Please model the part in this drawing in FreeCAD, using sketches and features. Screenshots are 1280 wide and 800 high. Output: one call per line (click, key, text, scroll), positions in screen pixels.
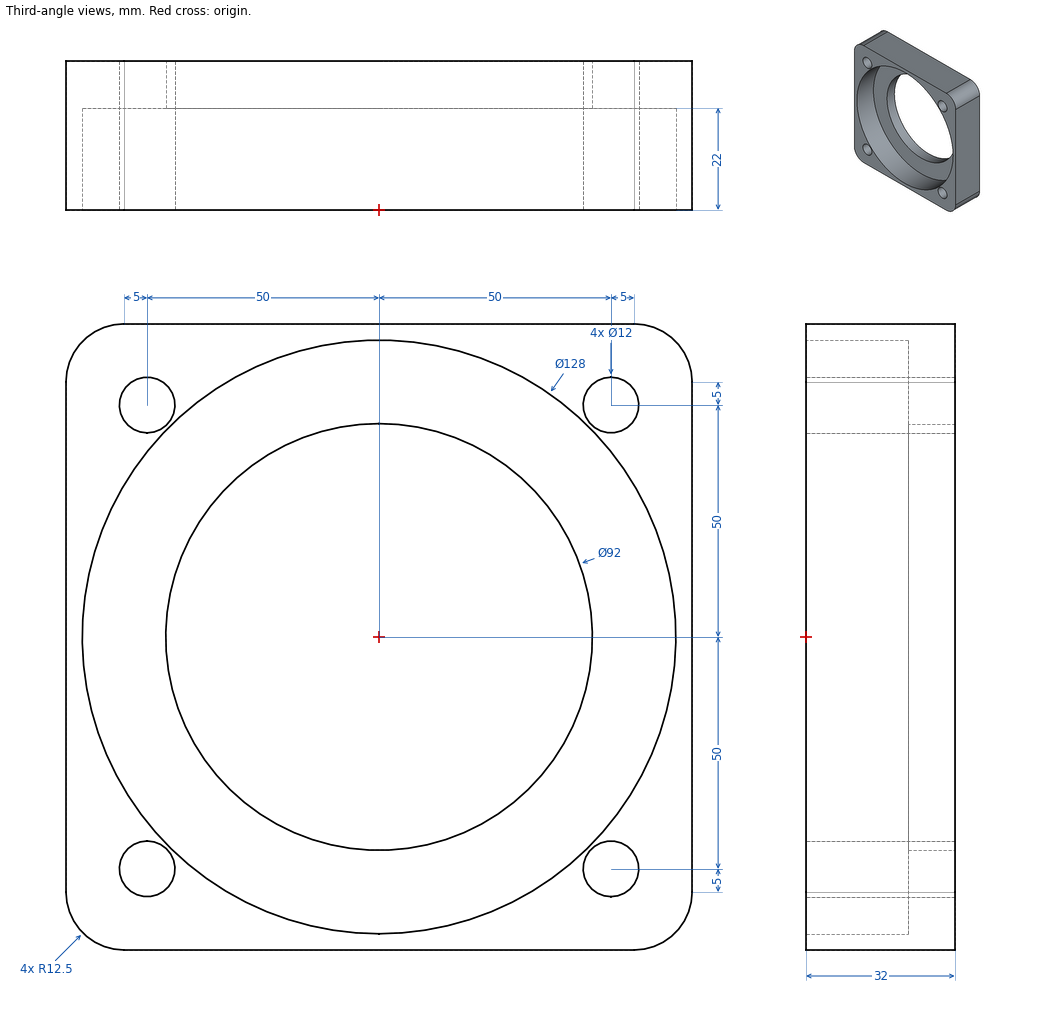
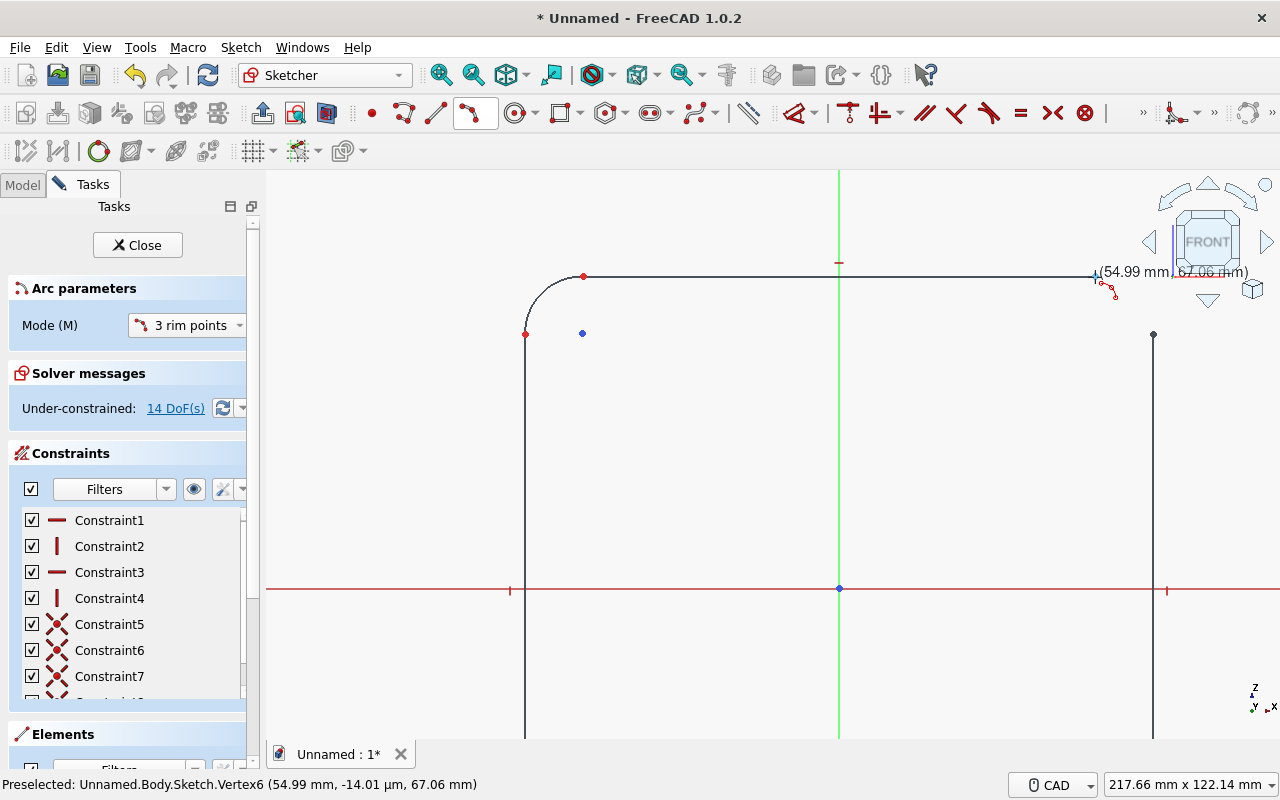
scroll(541, 291, down, 3)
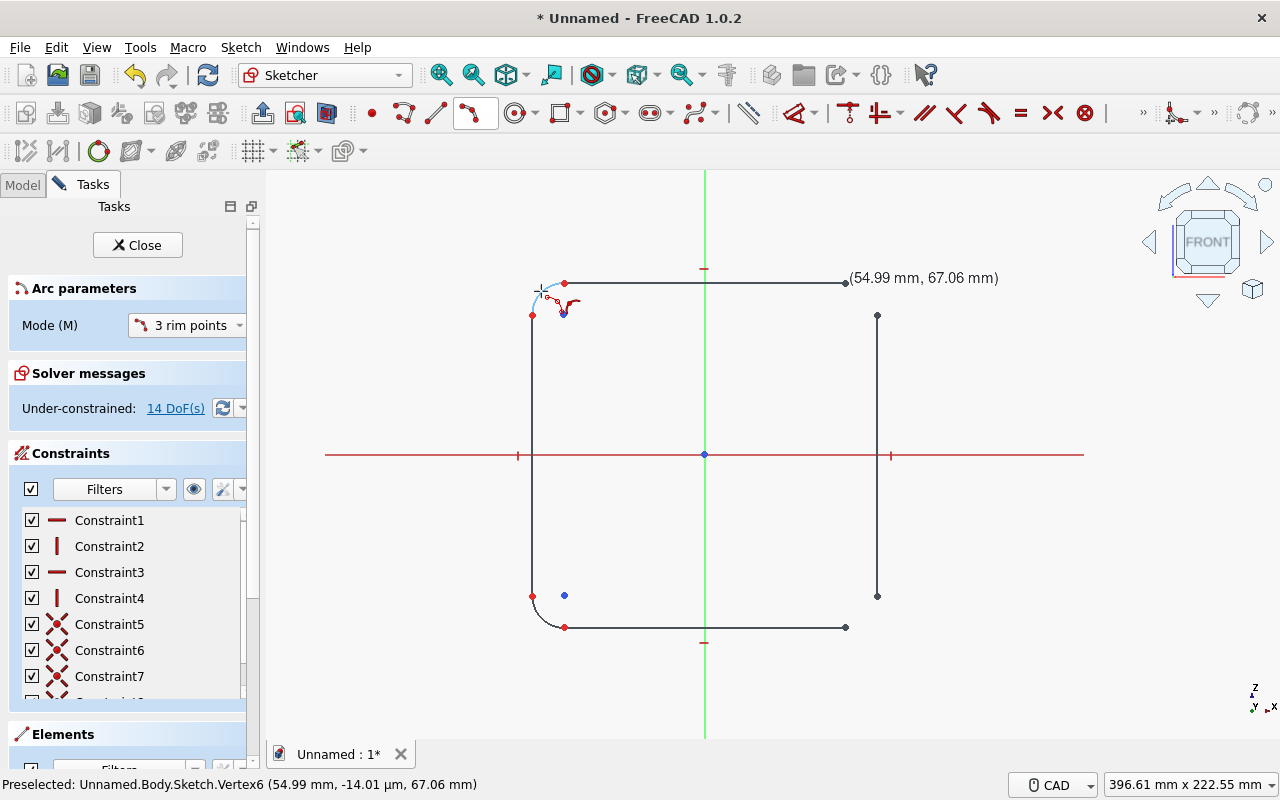
click(877, 315)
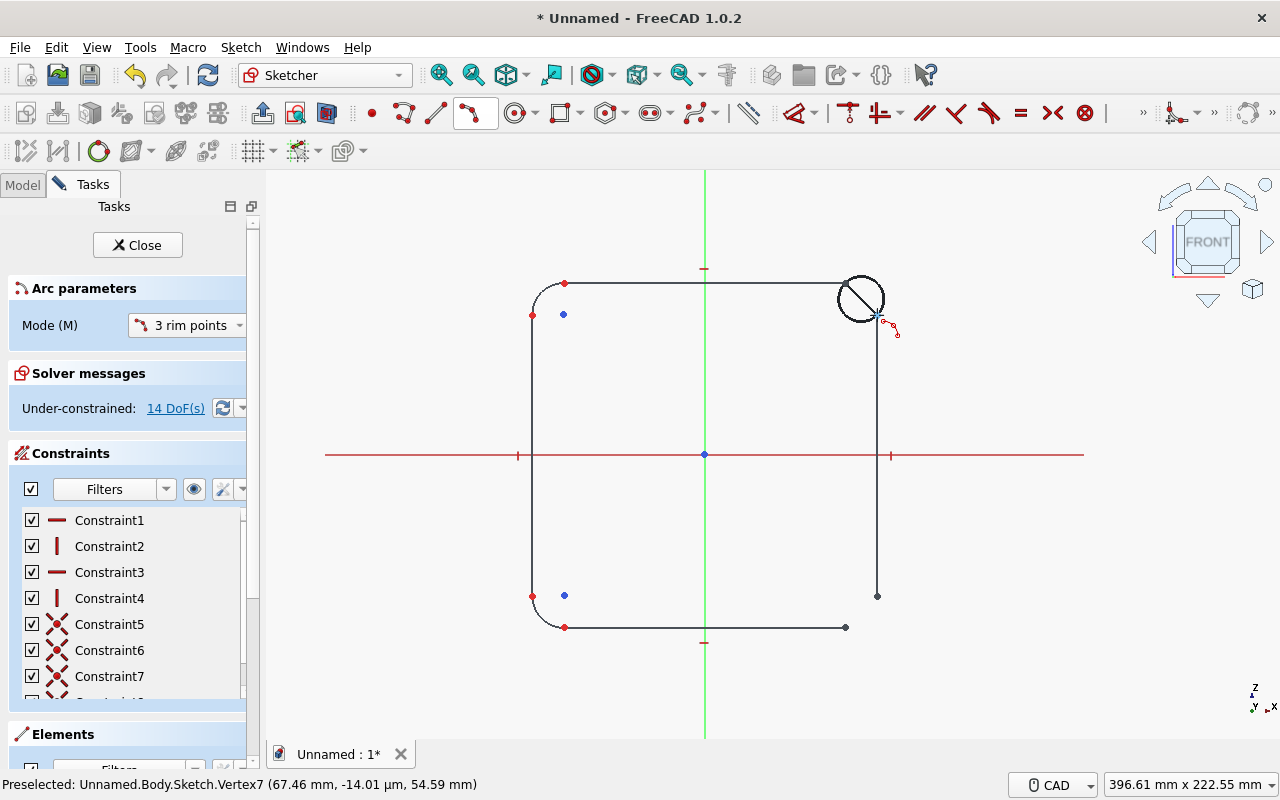
scroll(868, 291, up, 3)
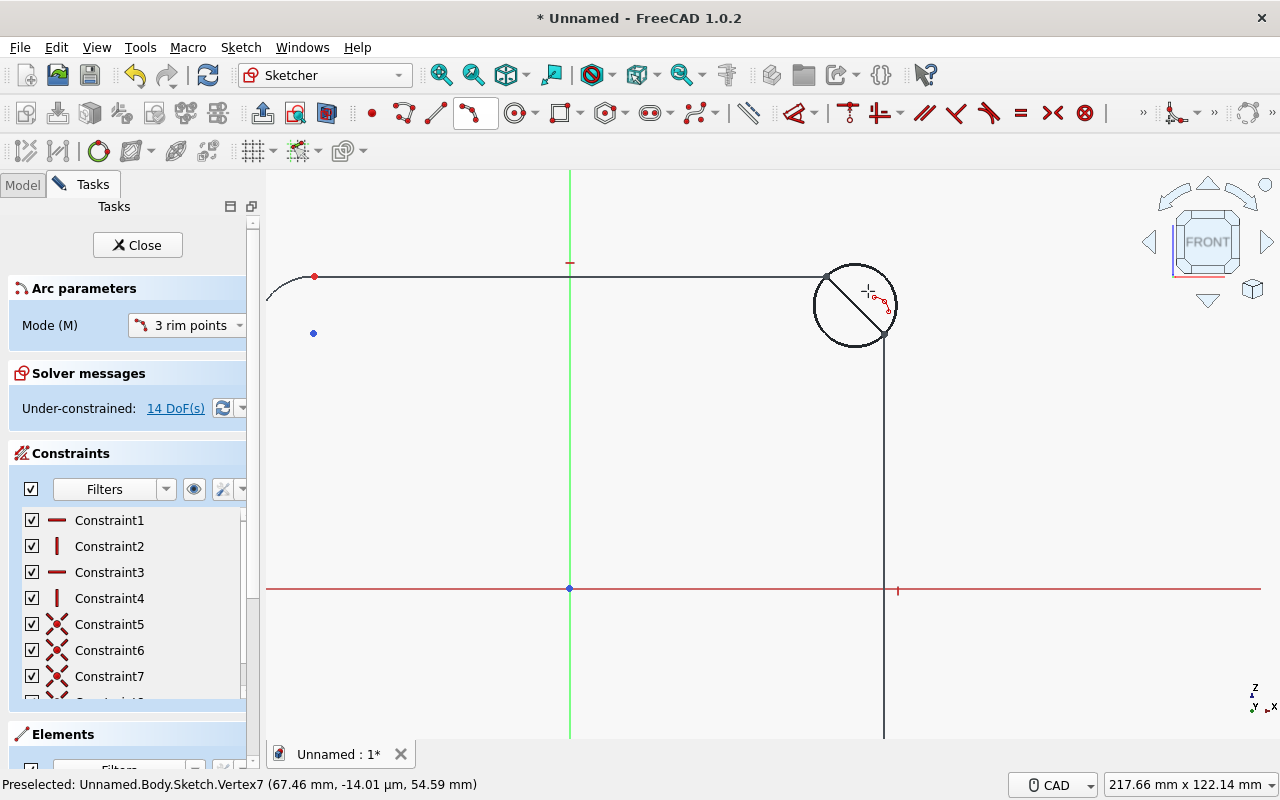
click(867, 292)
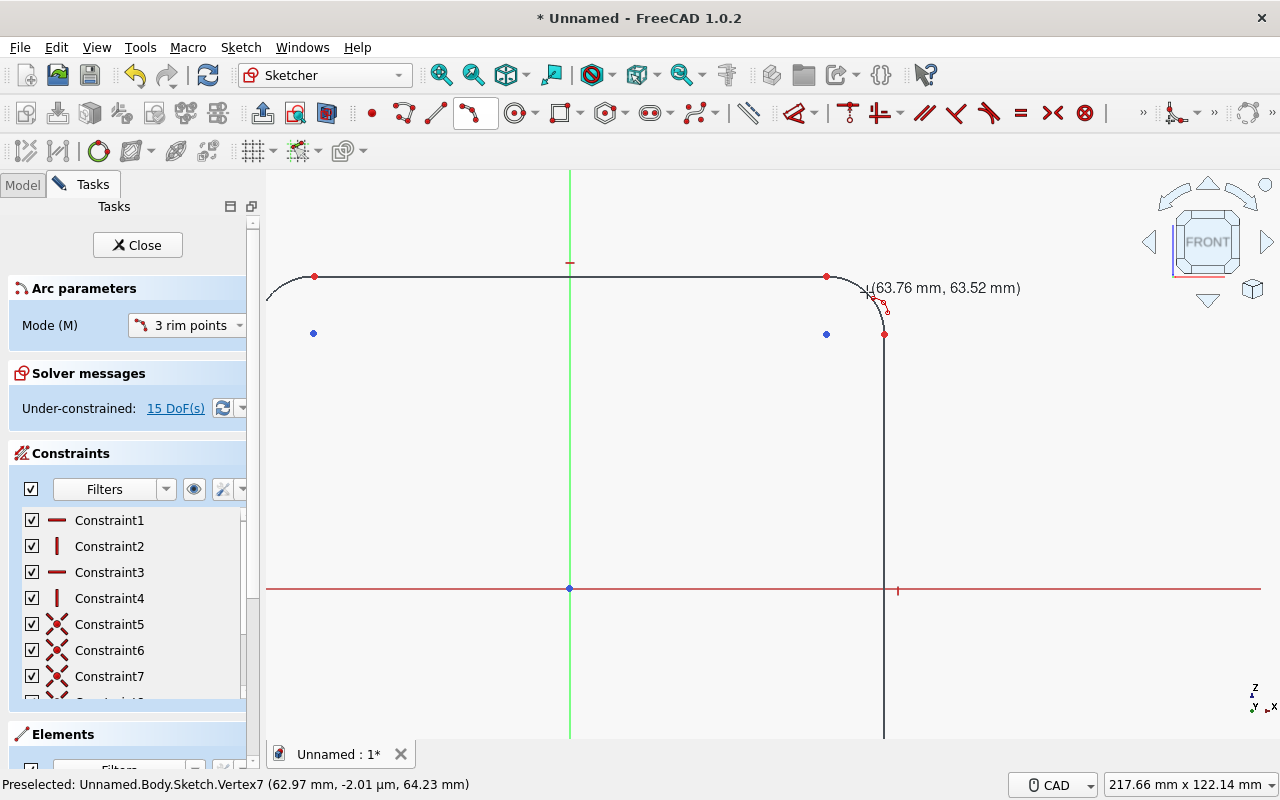
scroll(868, 291, down, 3)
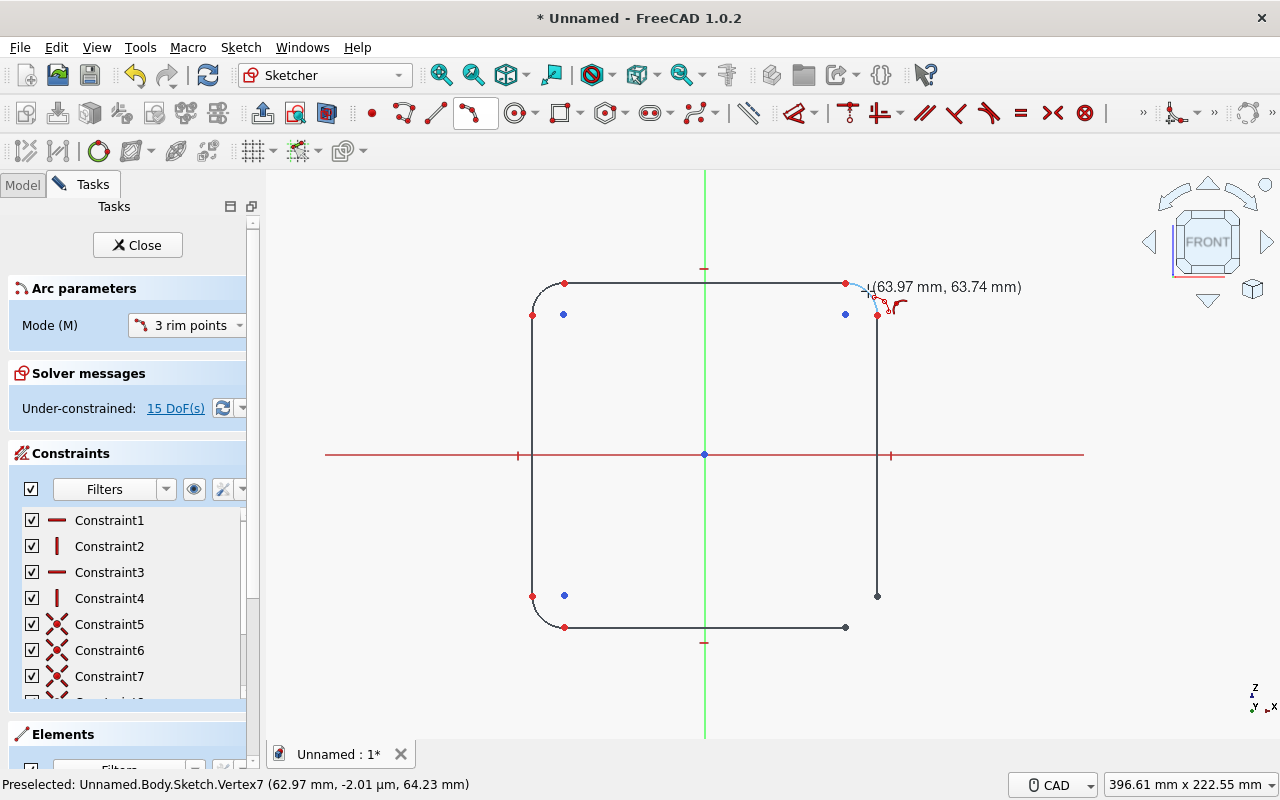
click(877, 596)
click(845, 628)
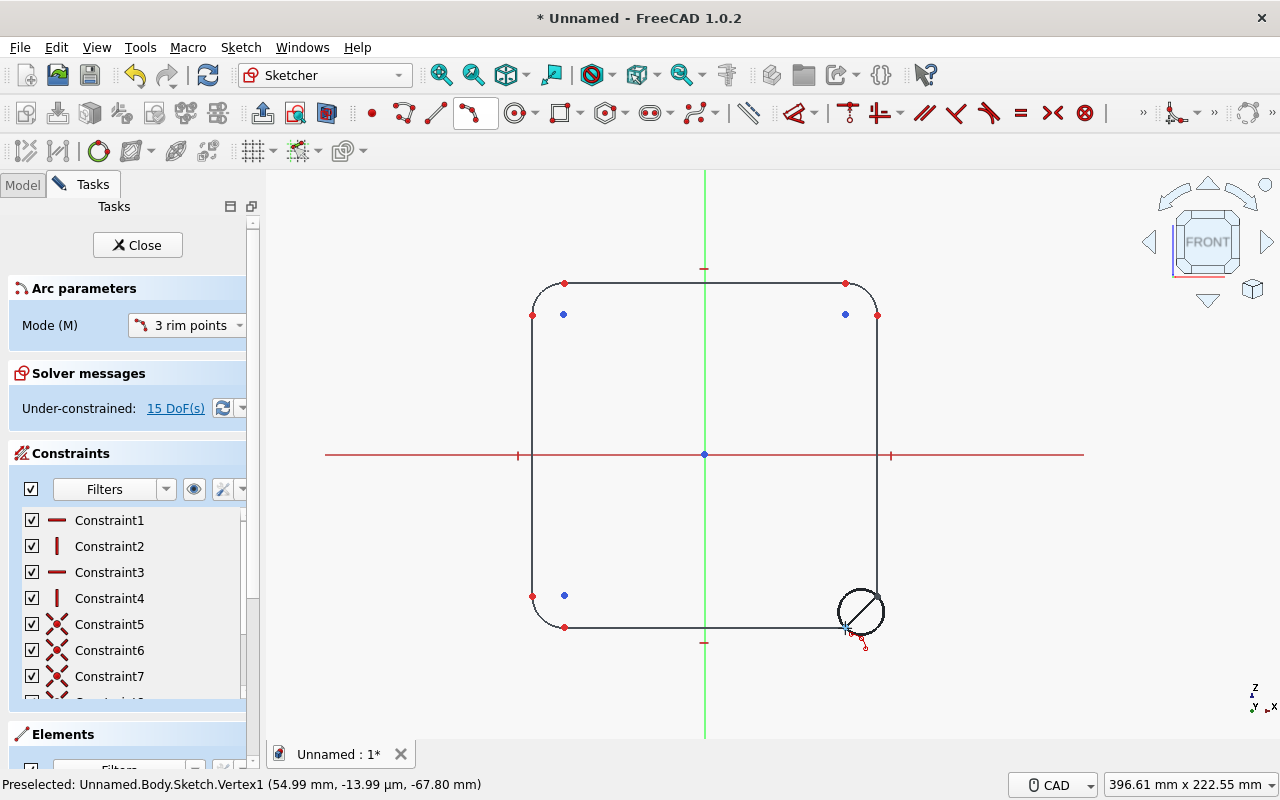
scroll(868, 618, up, 3)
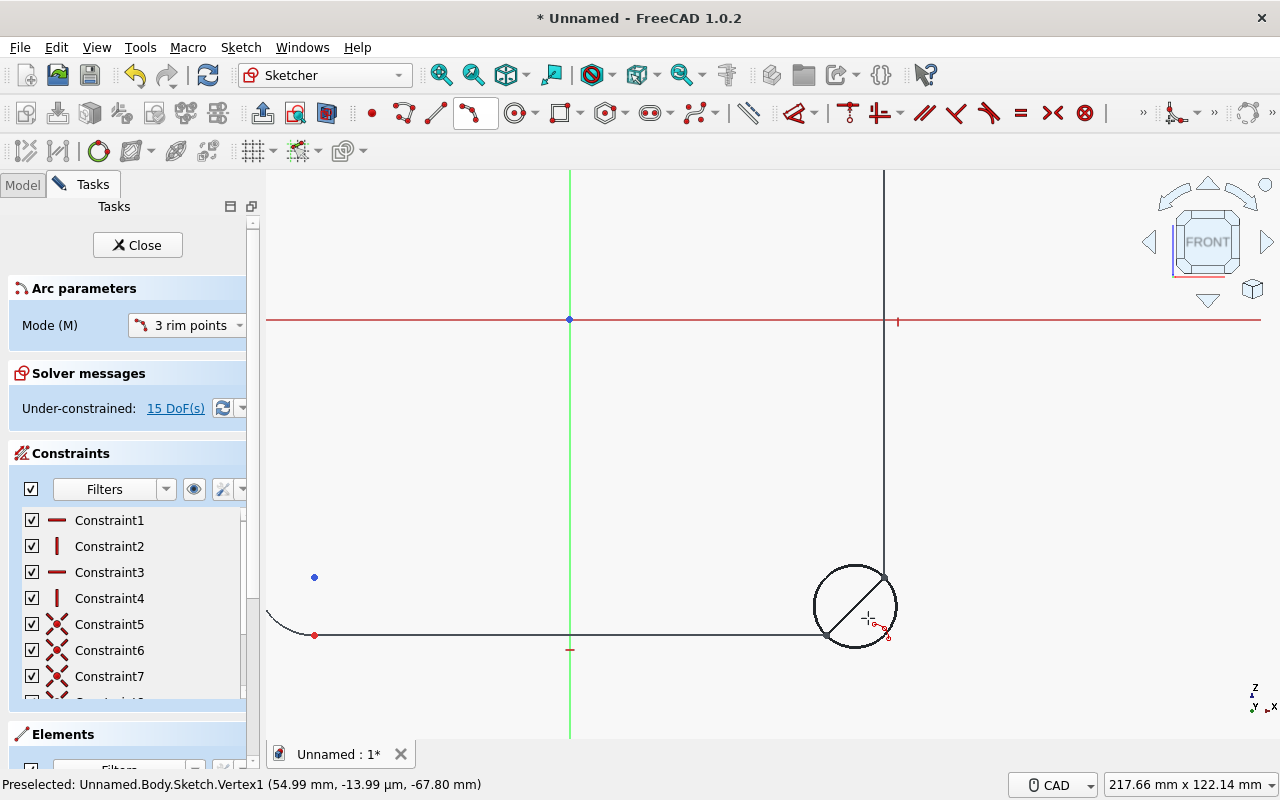
click(867, 617)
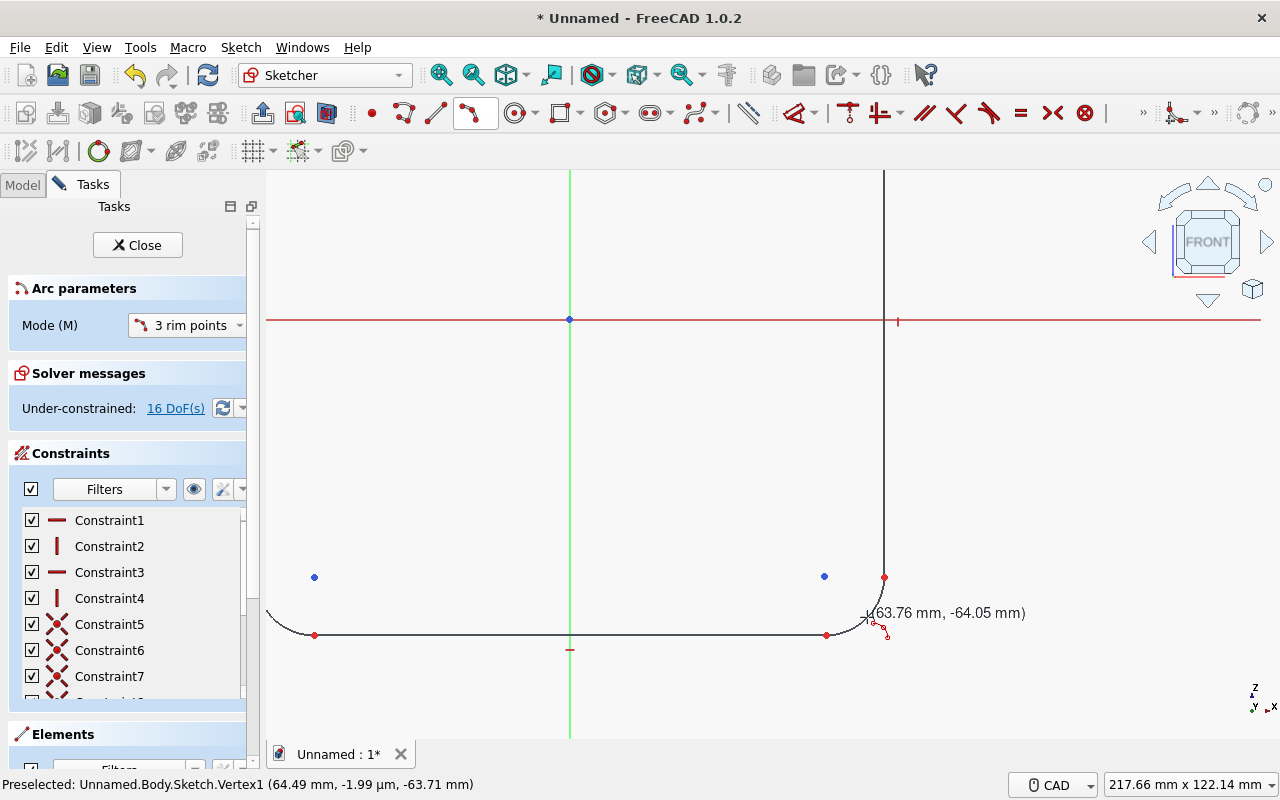
click(516, 114)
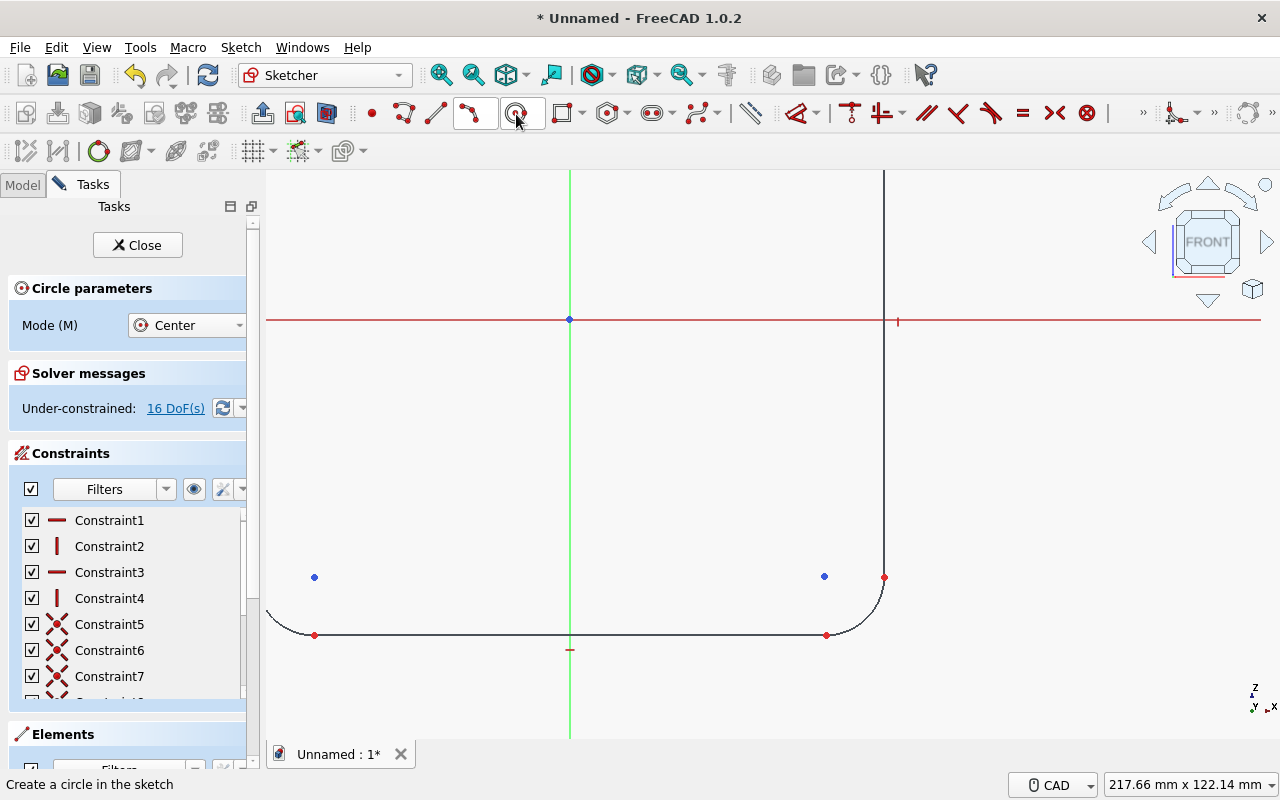
scroll(868, 619, down, 3)